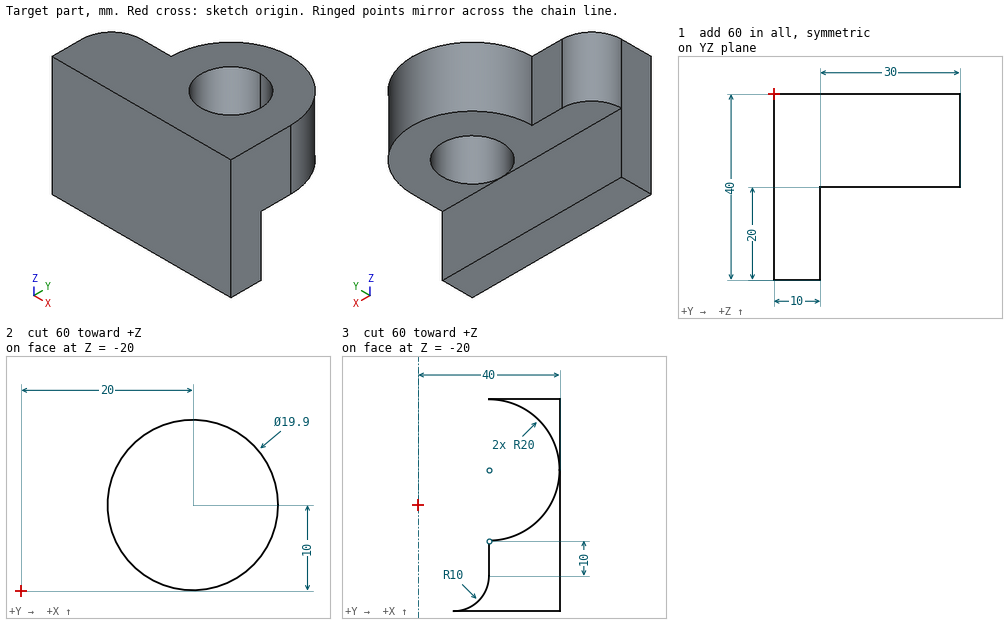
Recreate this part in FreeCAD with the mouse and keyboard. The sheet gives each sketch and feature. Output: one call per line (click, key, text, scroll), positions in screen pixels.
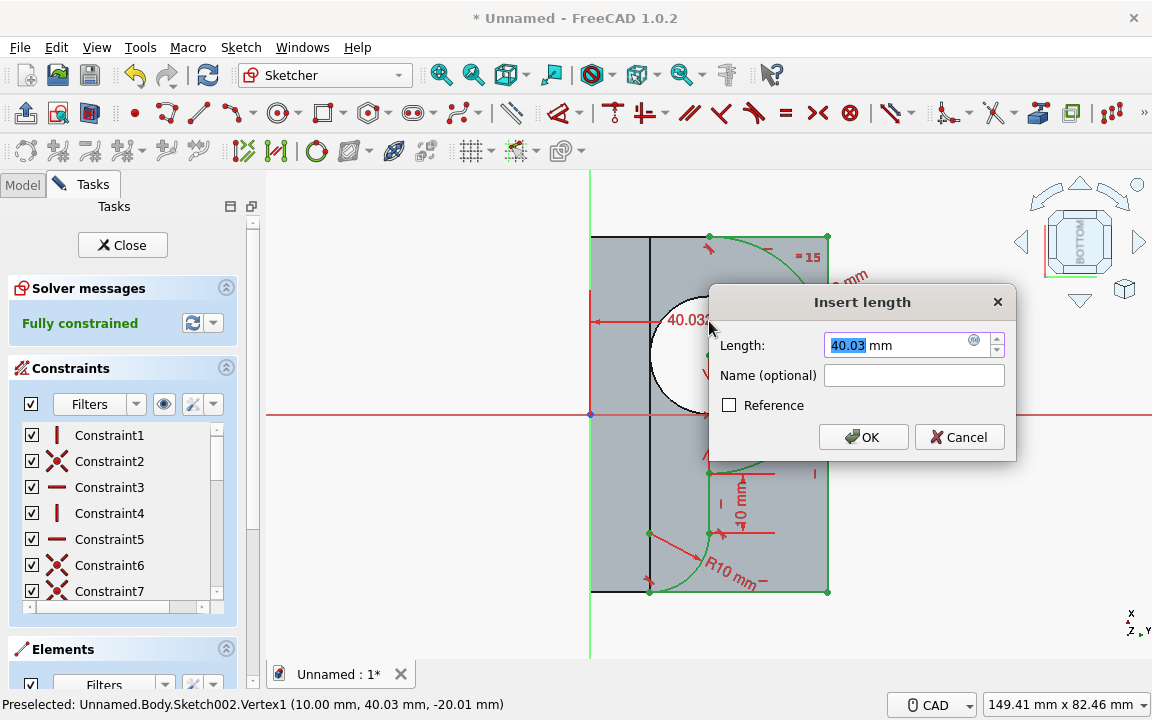
text(40)
key(Return)
key(Escape)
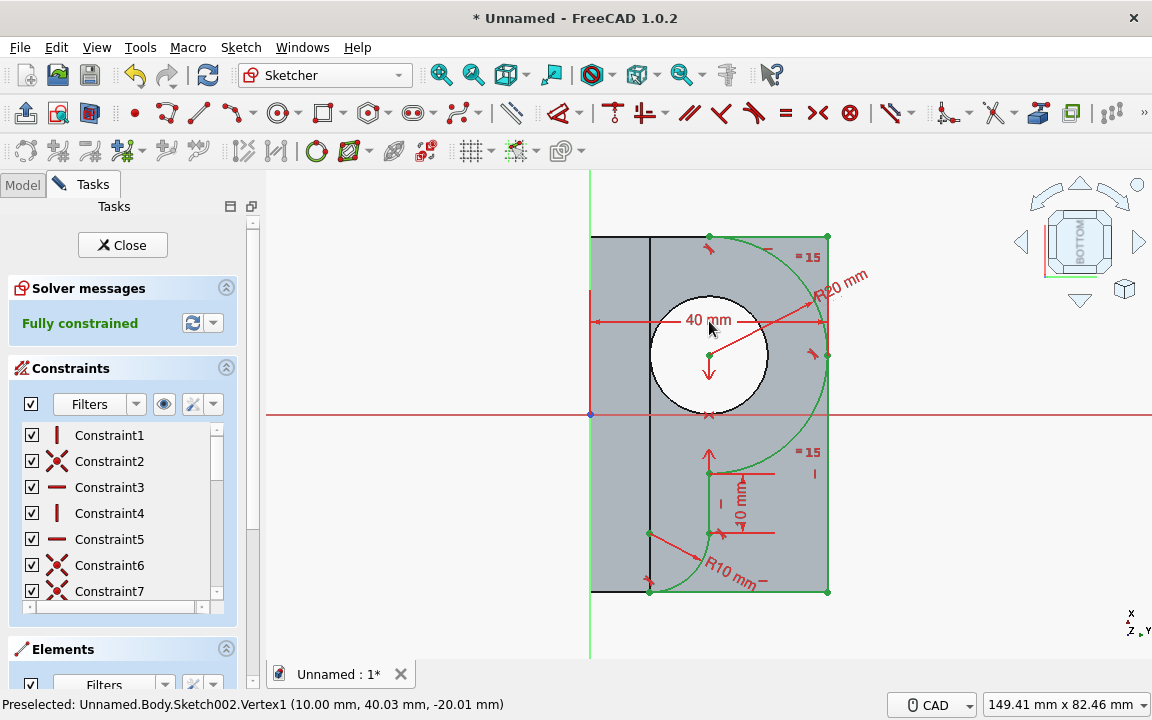
click(123, 245)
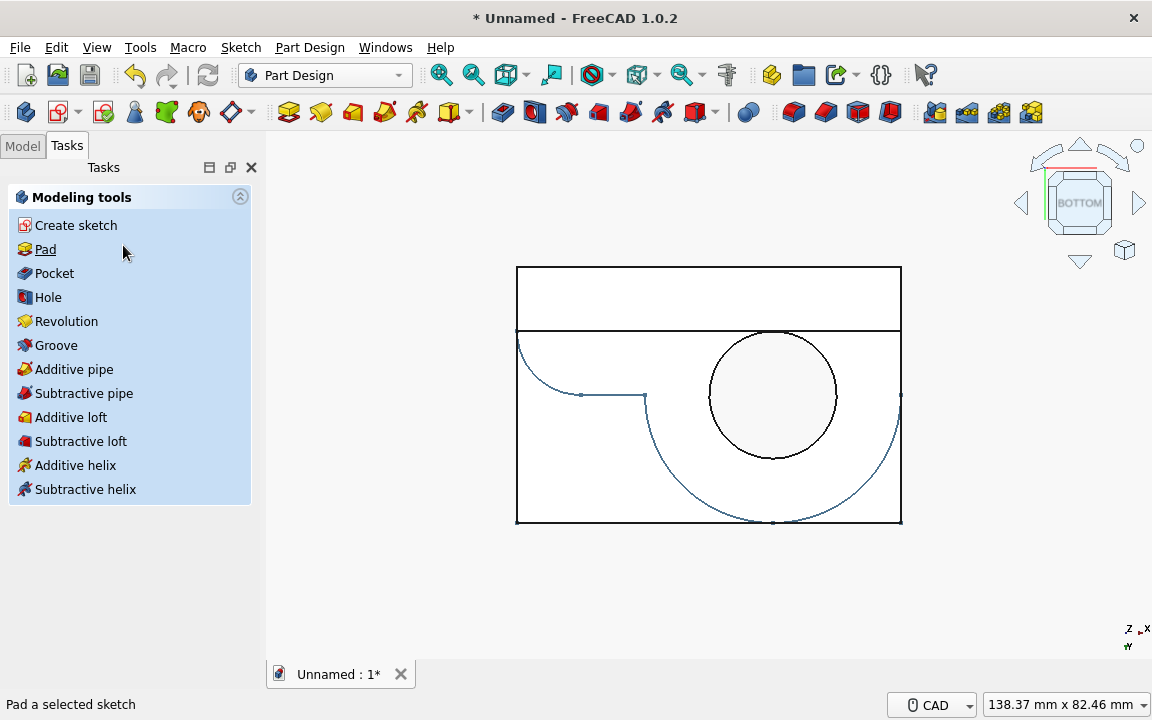
click(504, 112)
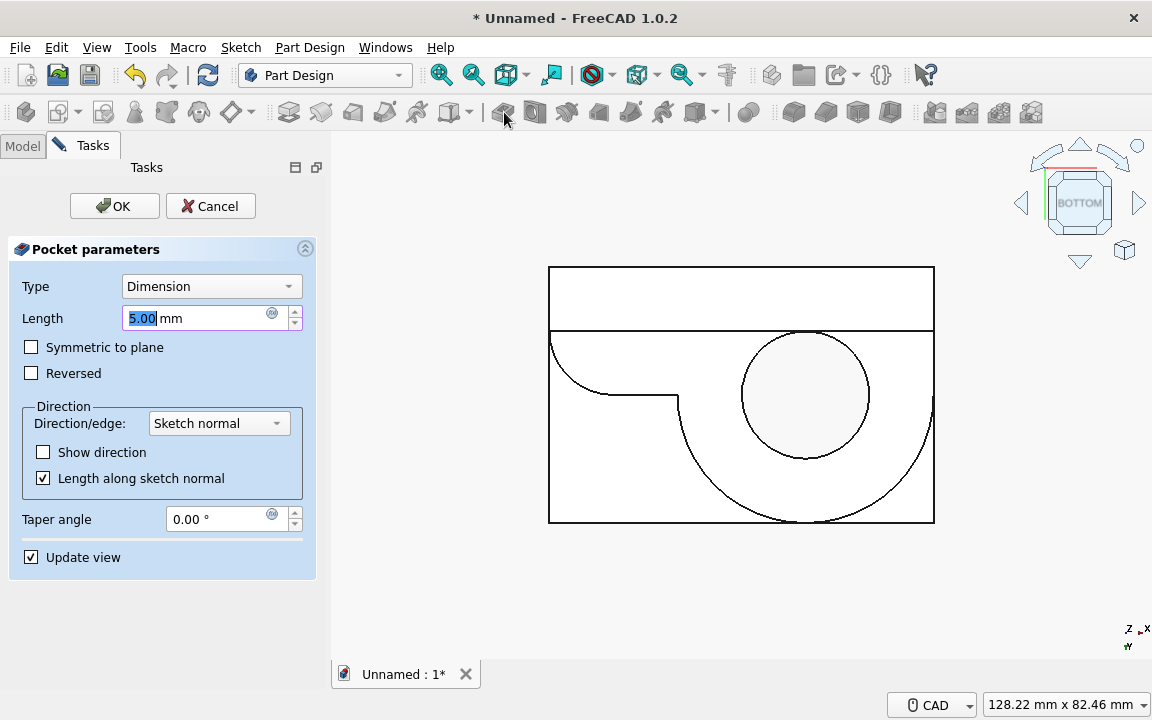
text(60)
key(Tab)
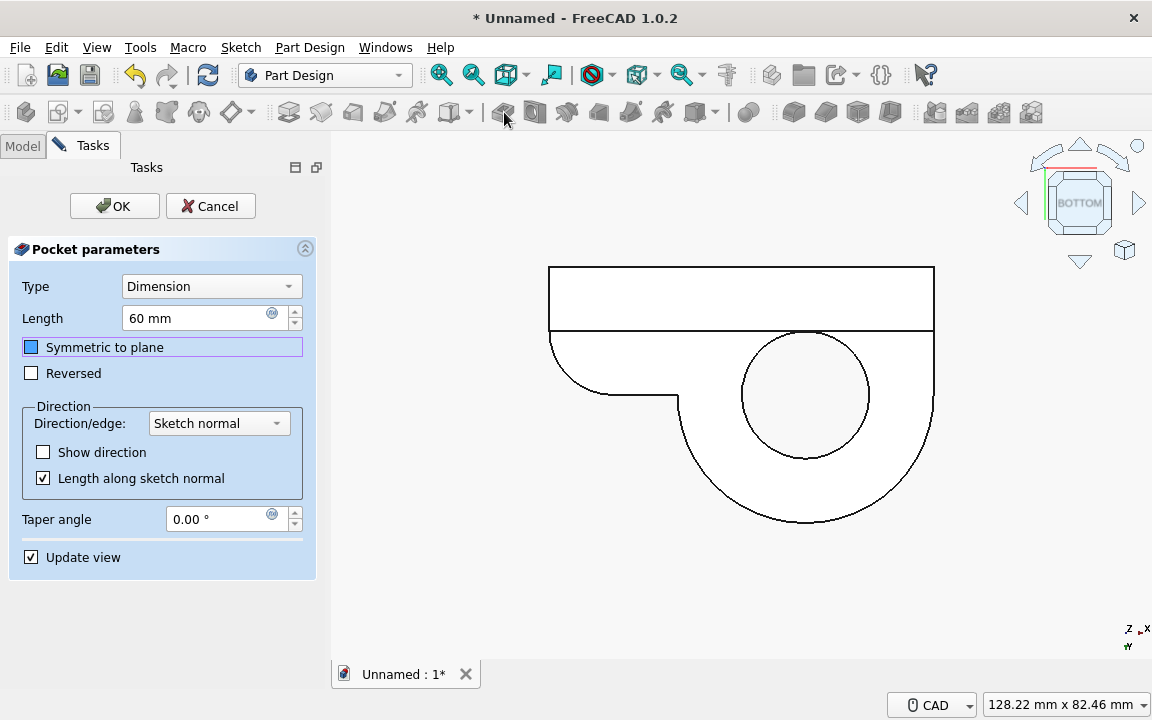
click(115, 206)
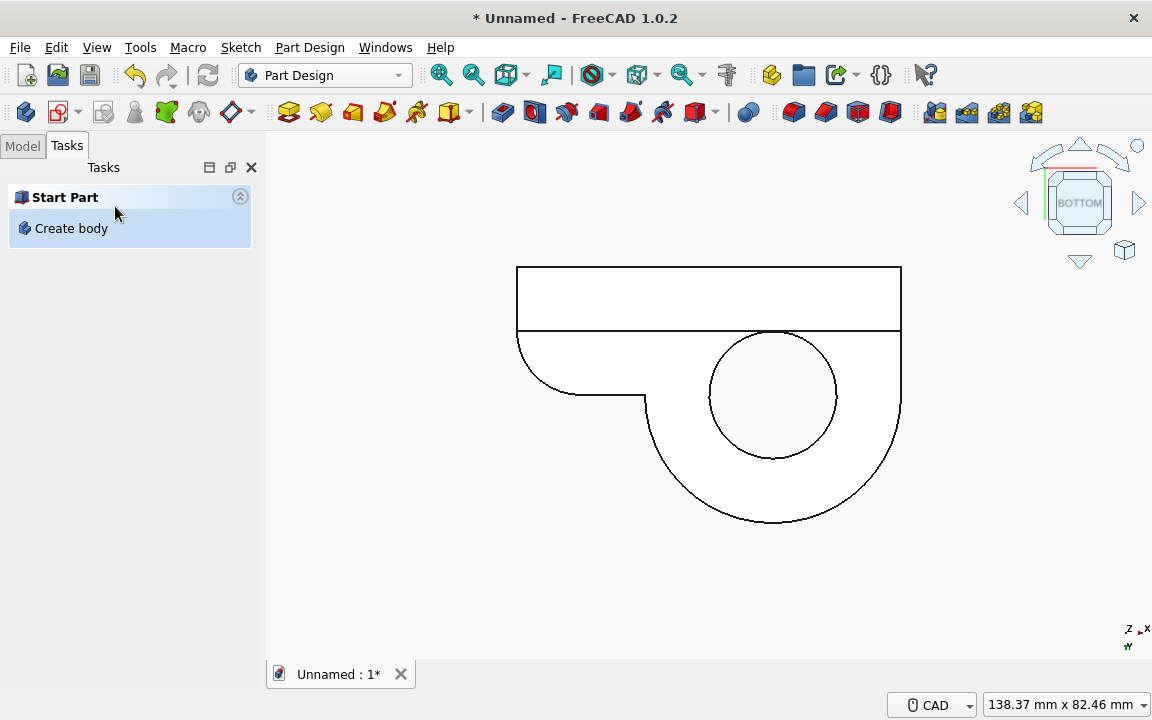
key(0)